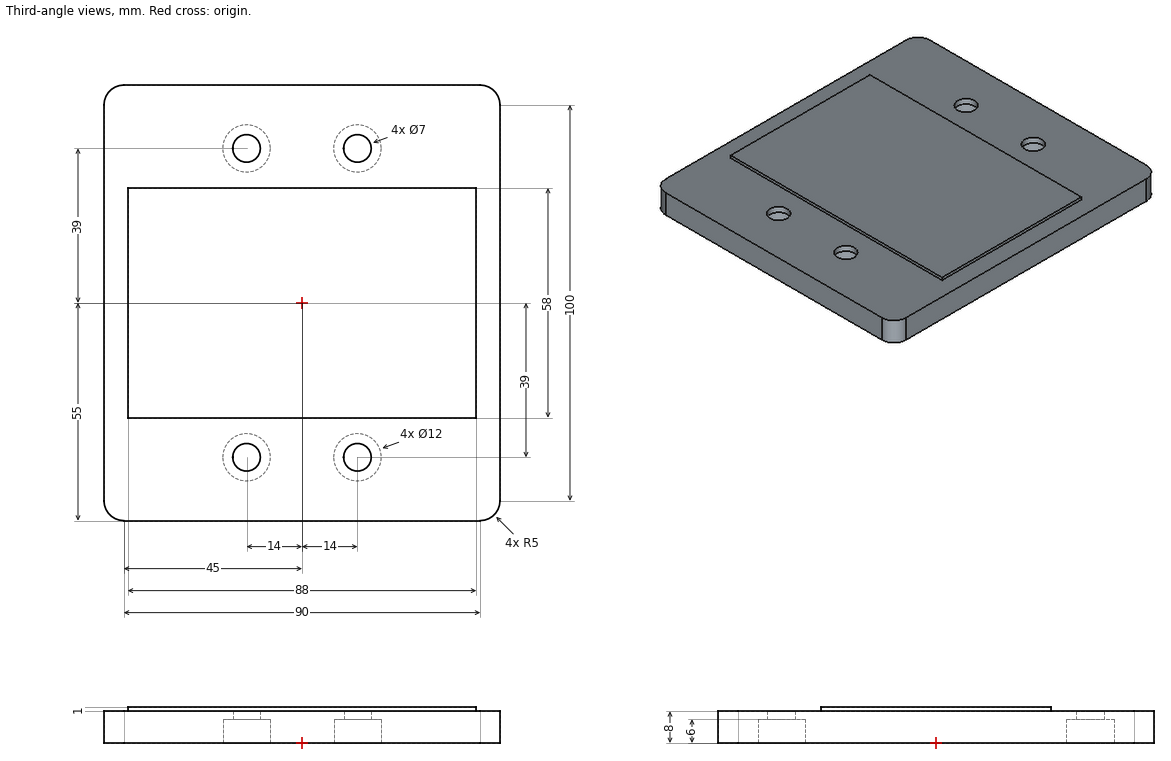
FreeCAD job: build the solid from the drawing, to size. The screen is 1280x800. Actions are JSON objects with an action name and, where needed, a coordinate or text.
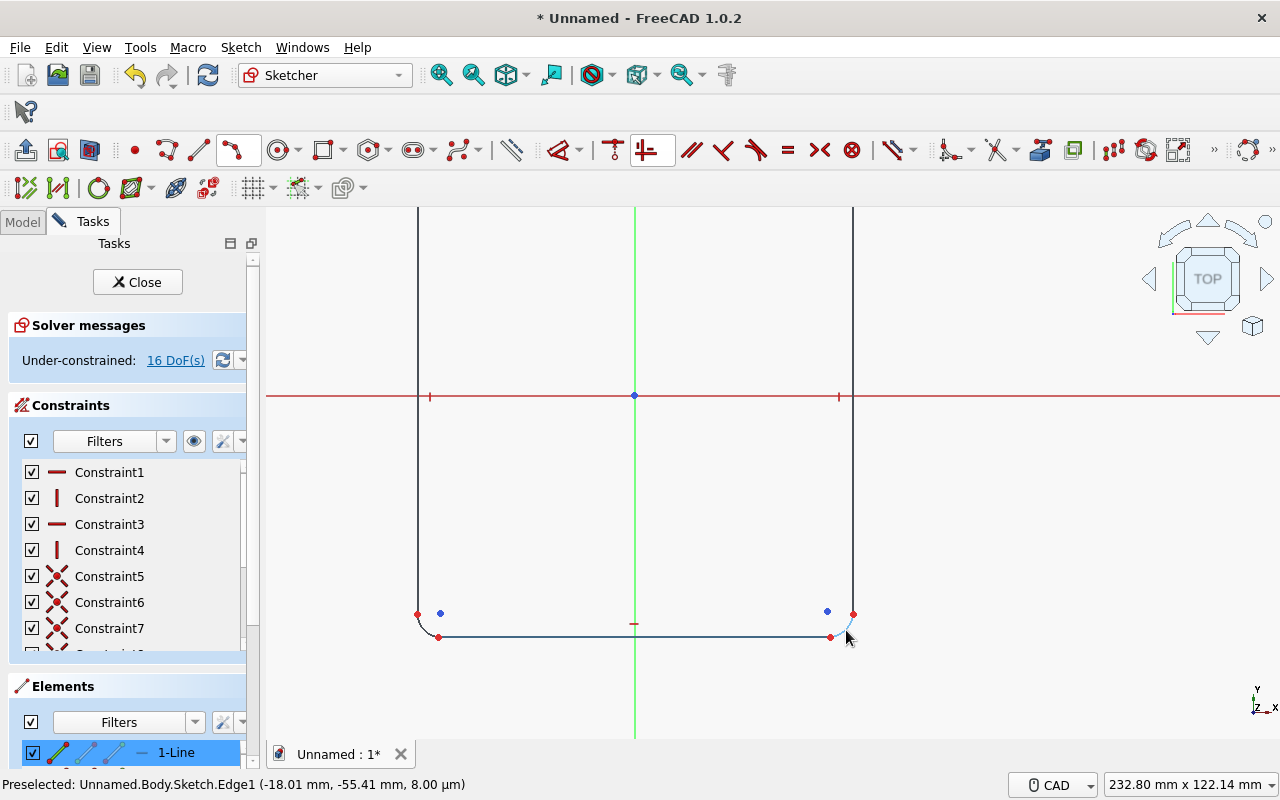
{"action": "left_click", "coordinate": [846, 630]}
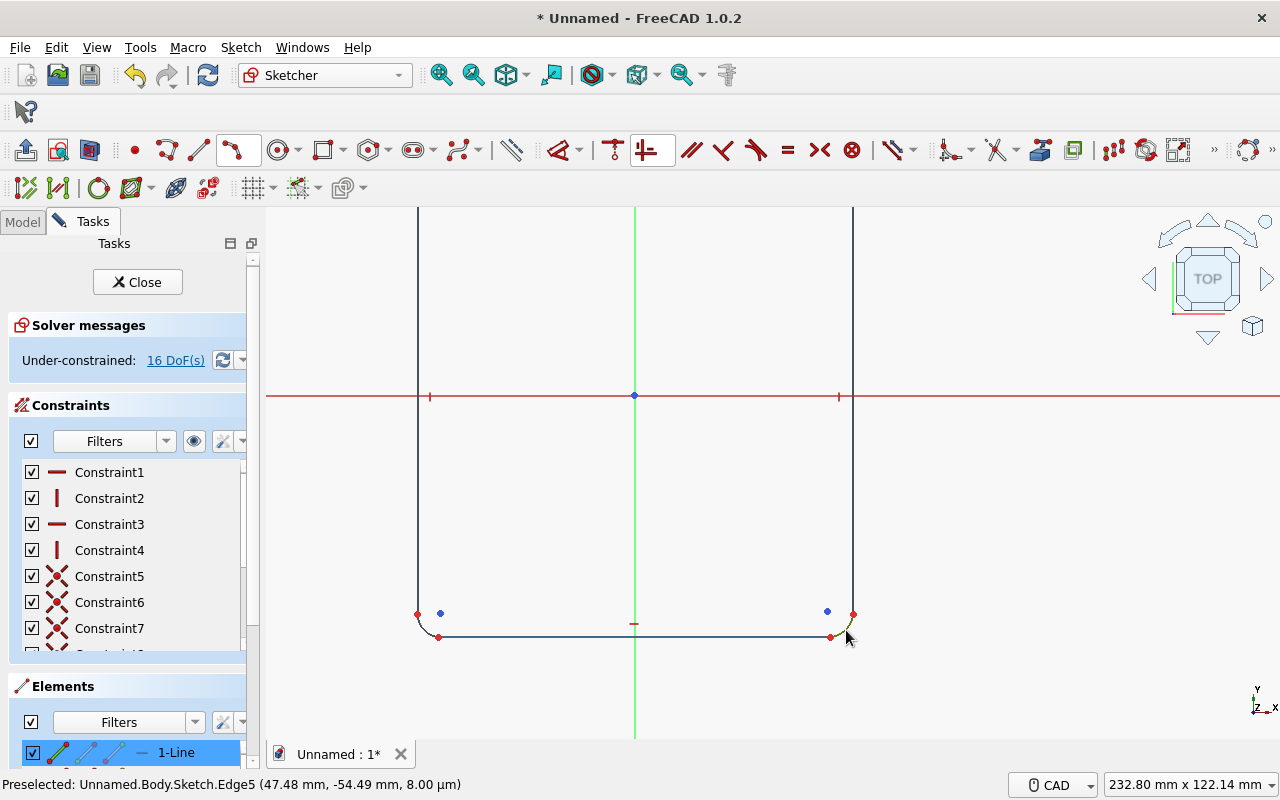
{"action": "left_click", "coordinate": [756, 150]}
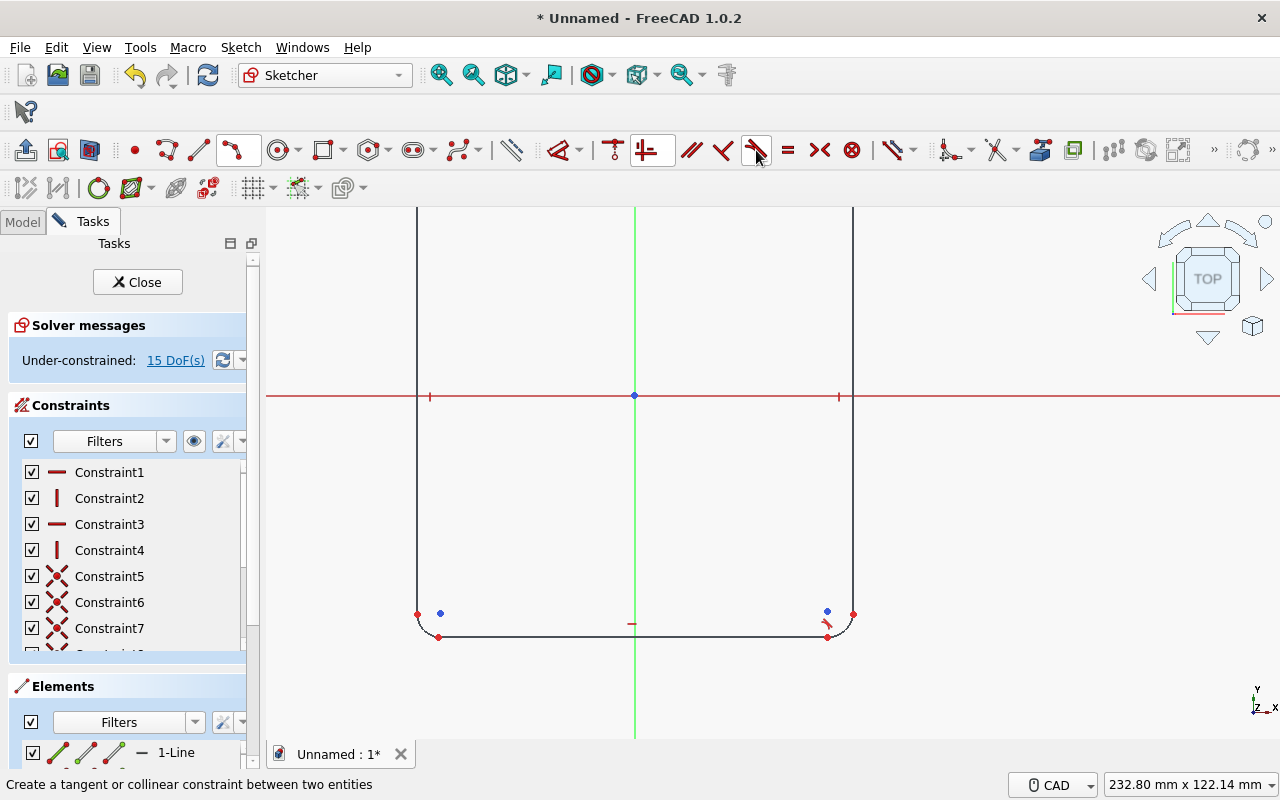
{"action": "left_click", "coordinate": [555, 637]}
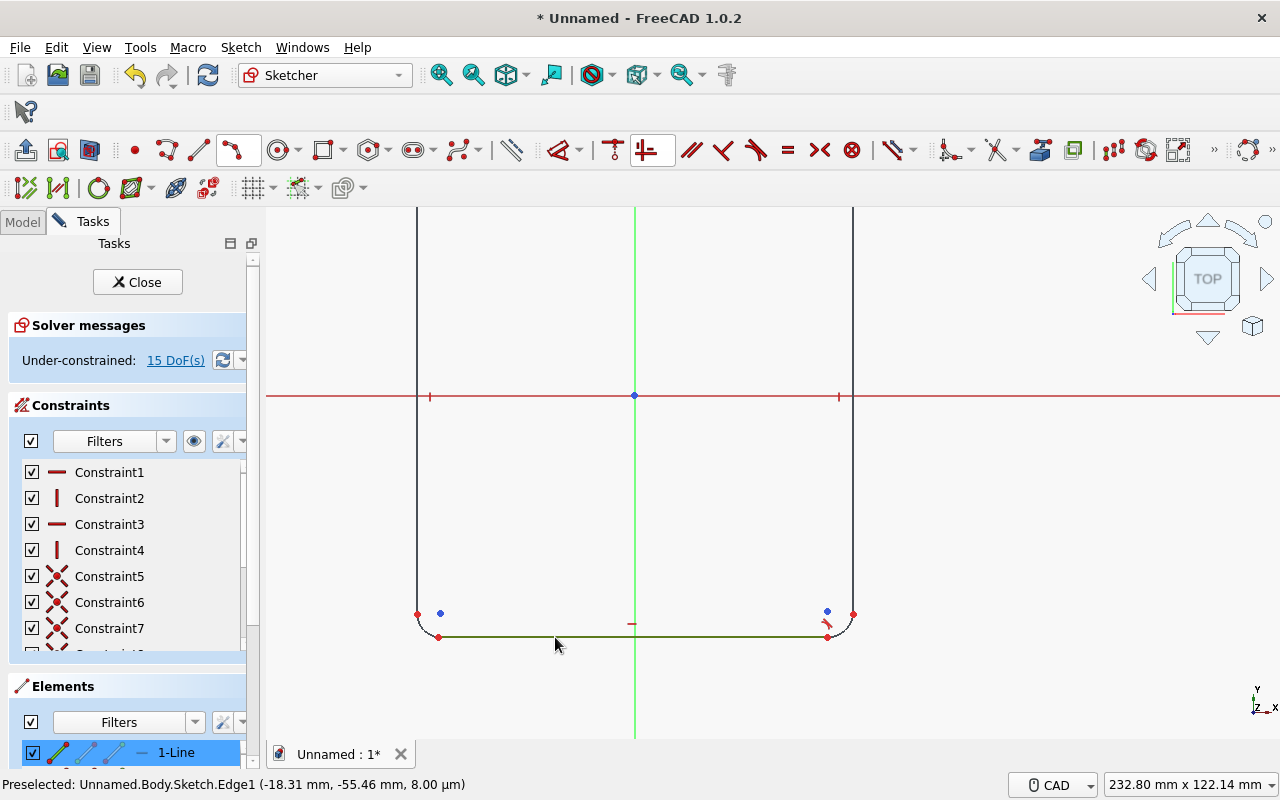
{"action": "scroll", "coordinate": [420, 624], "scroll_direction": "up", "scroll_amount": 2}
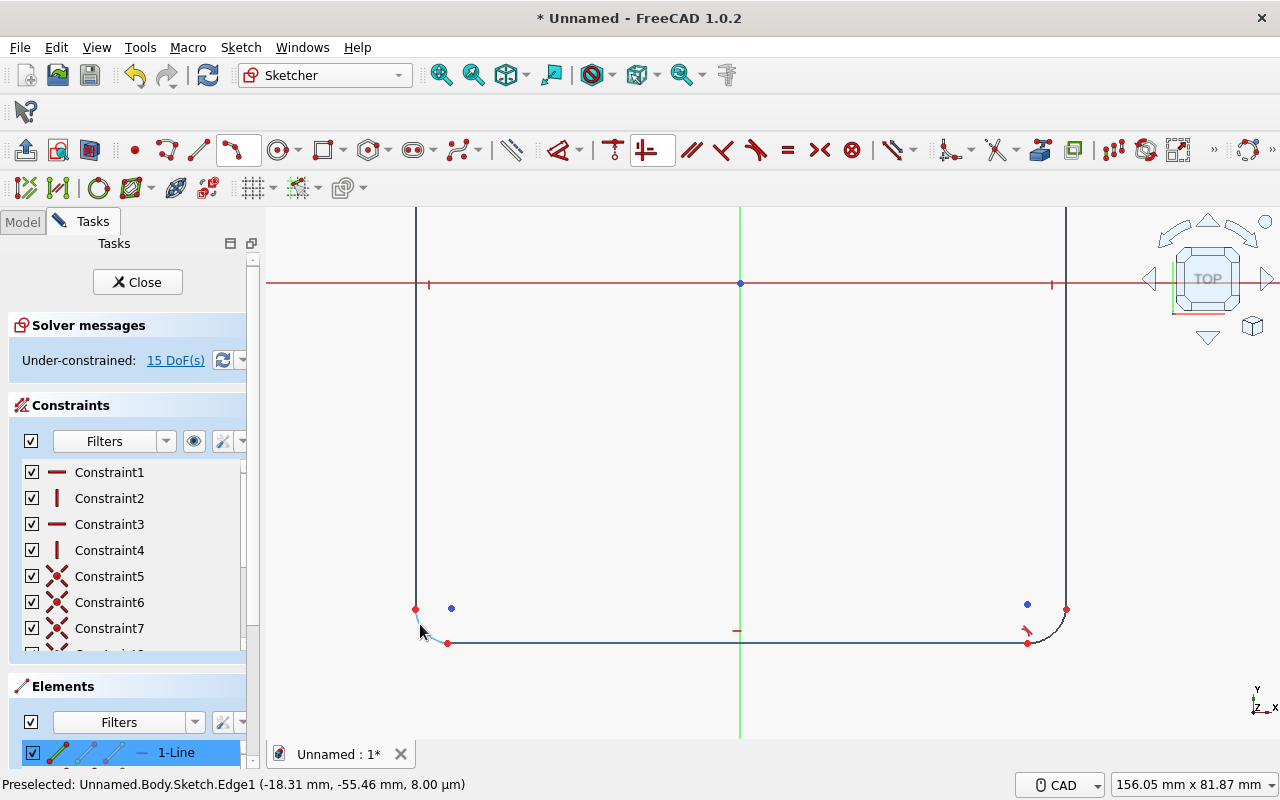
{"action": "left_click", "coordinate": [420, 624]}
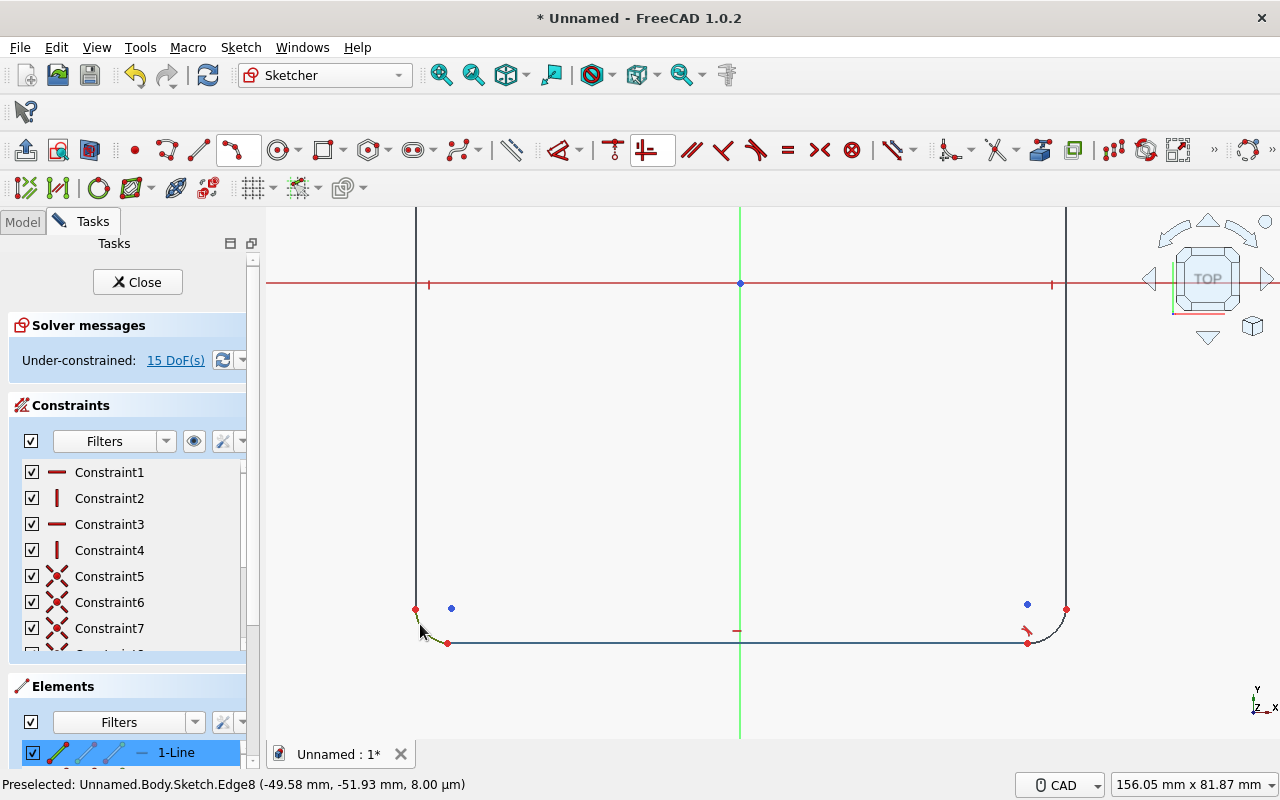
{"action": "key", "text": "t"}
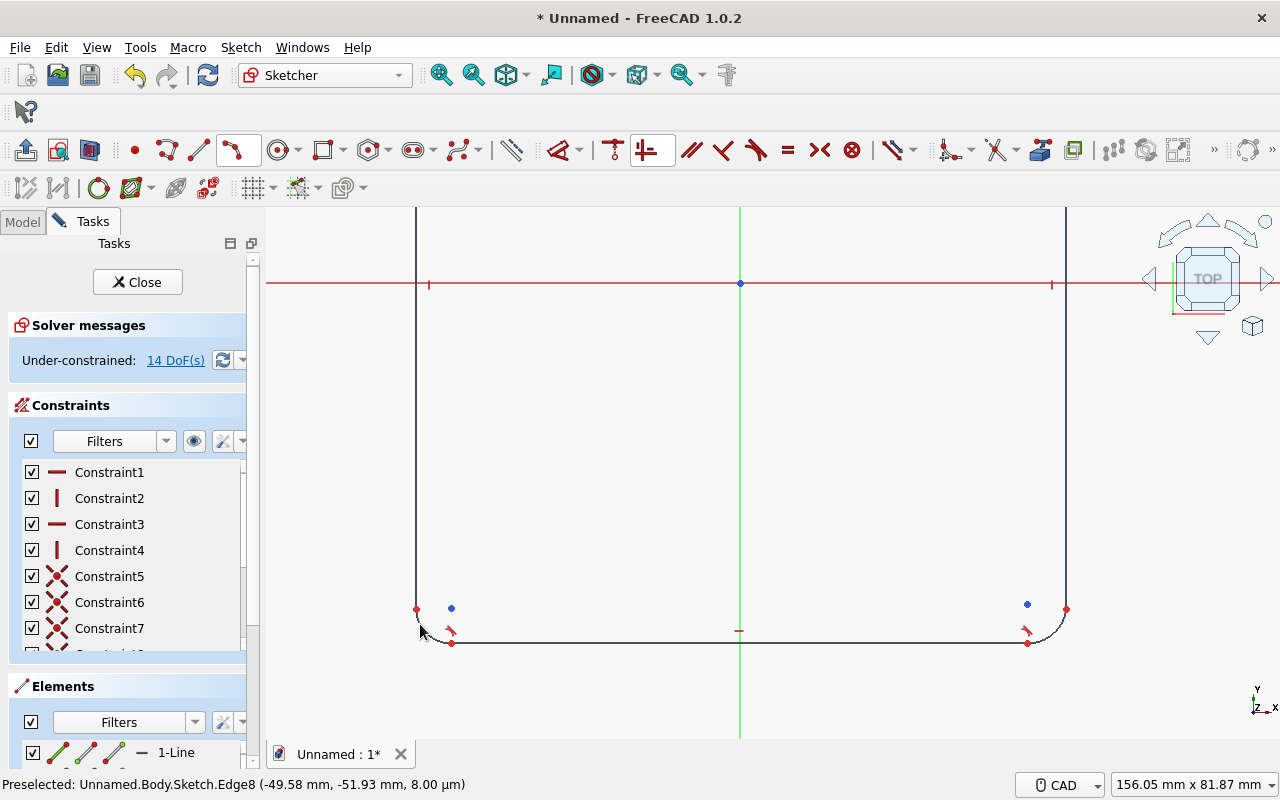
{"action": "left_click", "coordinate": [1066, 415]}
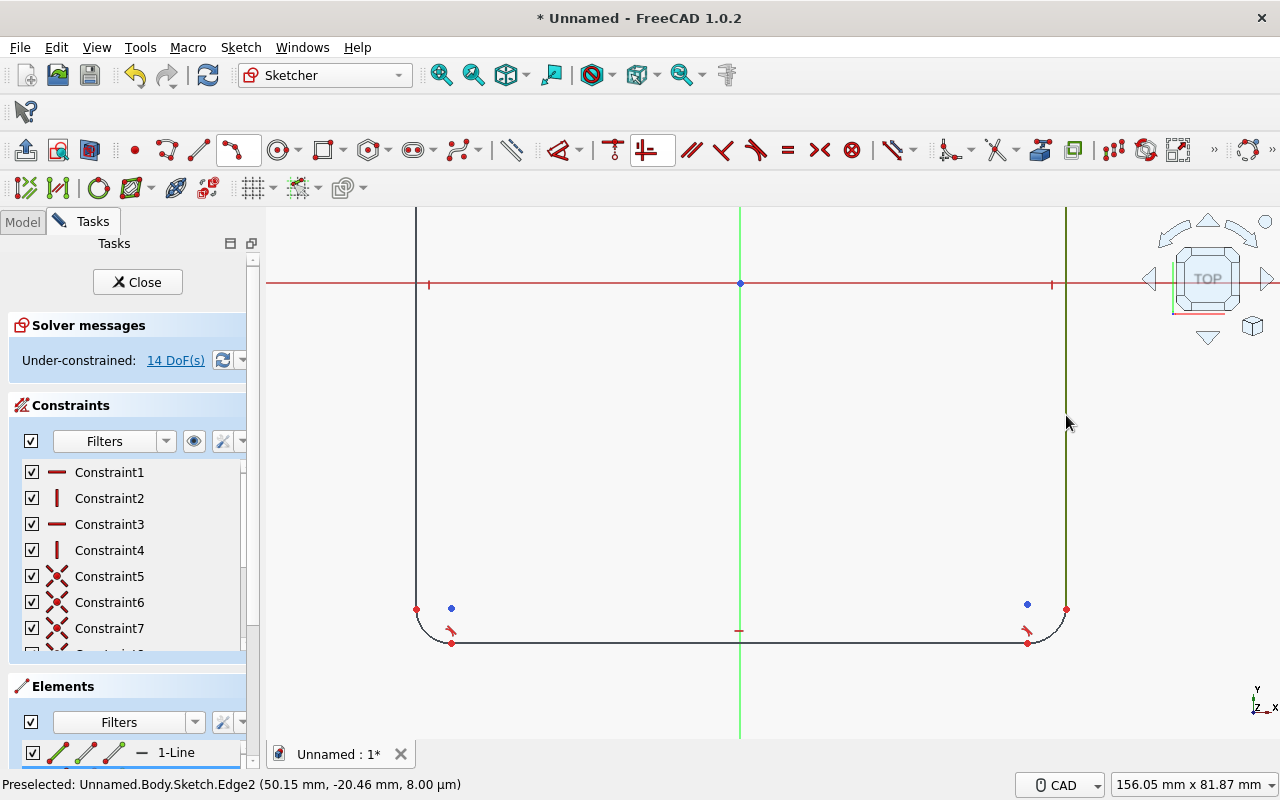
{"action": "left_click", "coordinate": [1044, 640]}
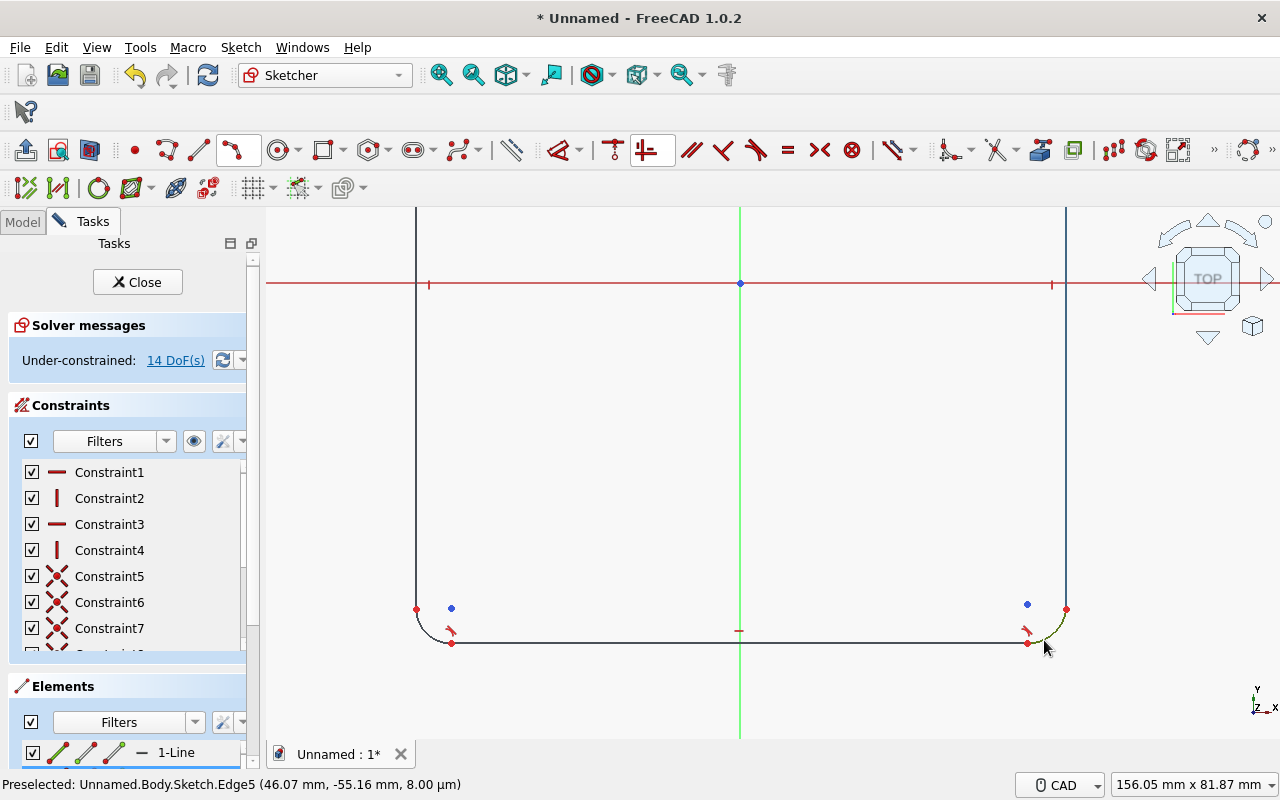
{"action": "left_click", "coordinate": [756, 150]}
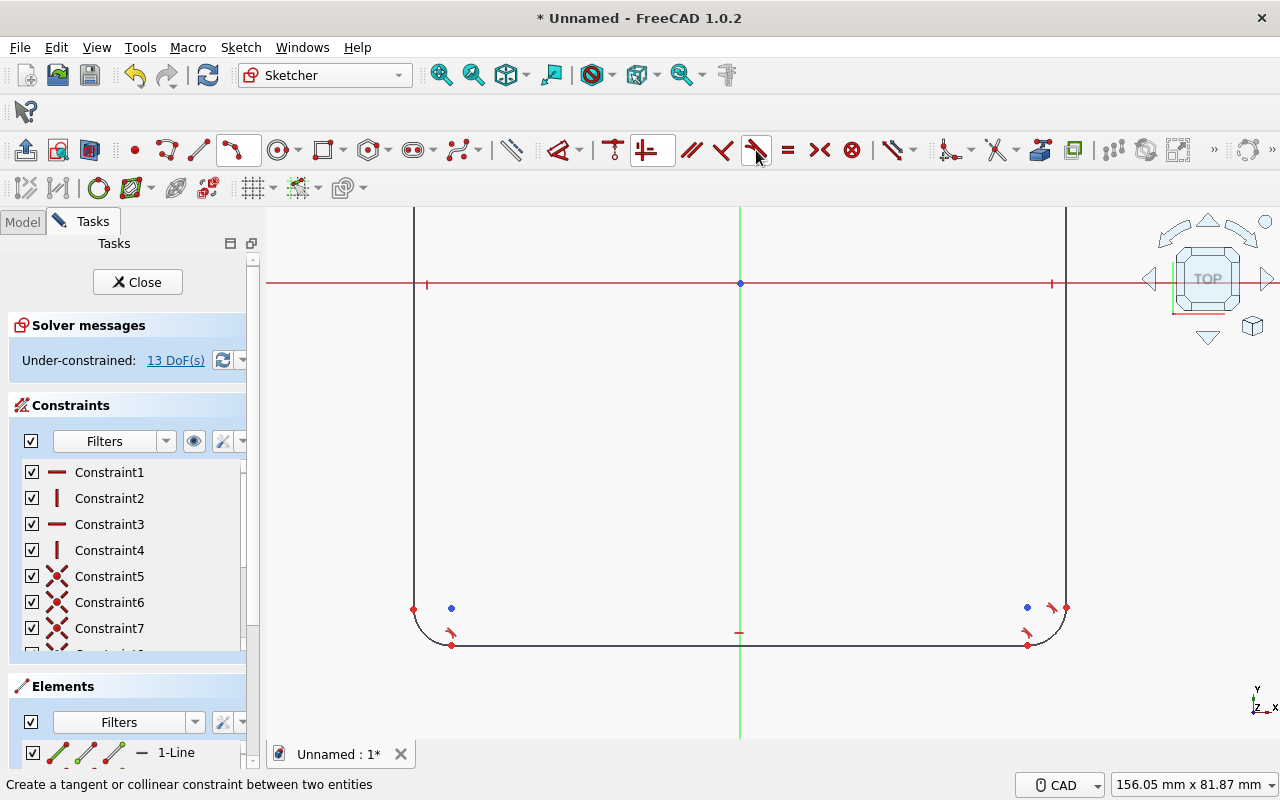
{"action": "left_click", "coordinate": [1066, 413]}